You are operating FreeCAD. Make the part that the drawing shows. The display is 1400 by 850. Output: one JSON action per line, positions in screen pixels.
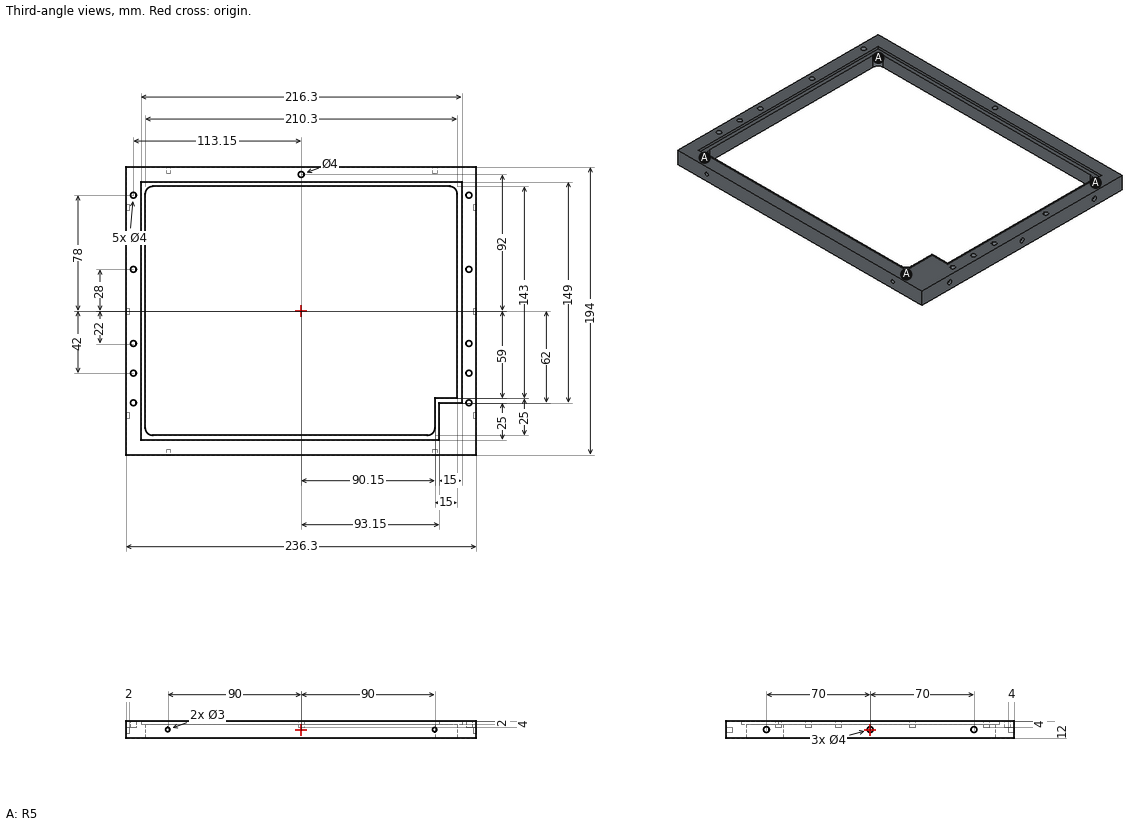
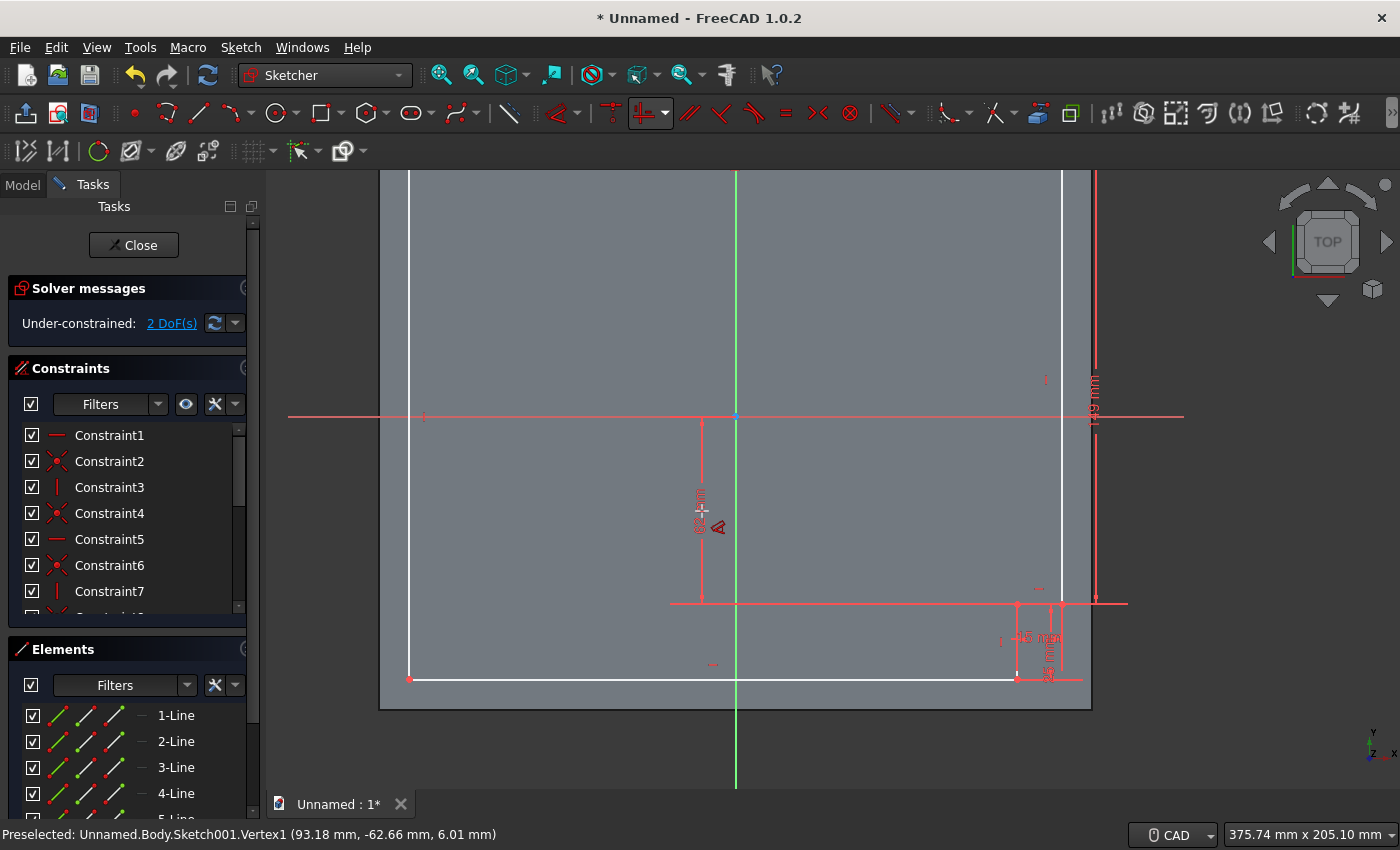
{"action": "scroll", "coordinate": [894, 761], "scroll_direction": "down", "scroll_amount": 1}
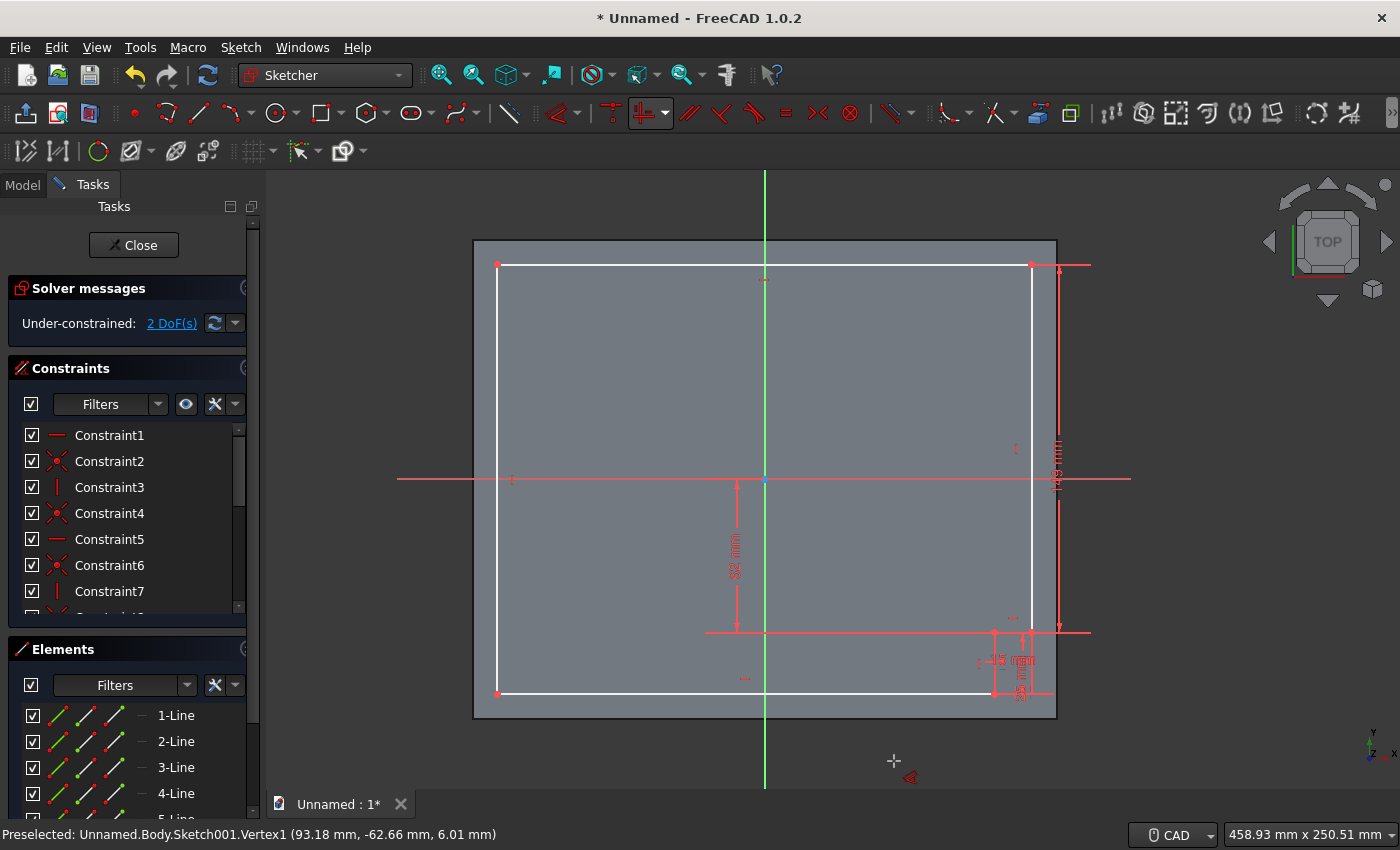
{"action": "left_click", "coordinate": [871, 265]}
{"action": "left_click", "coordinate": [641, 231]}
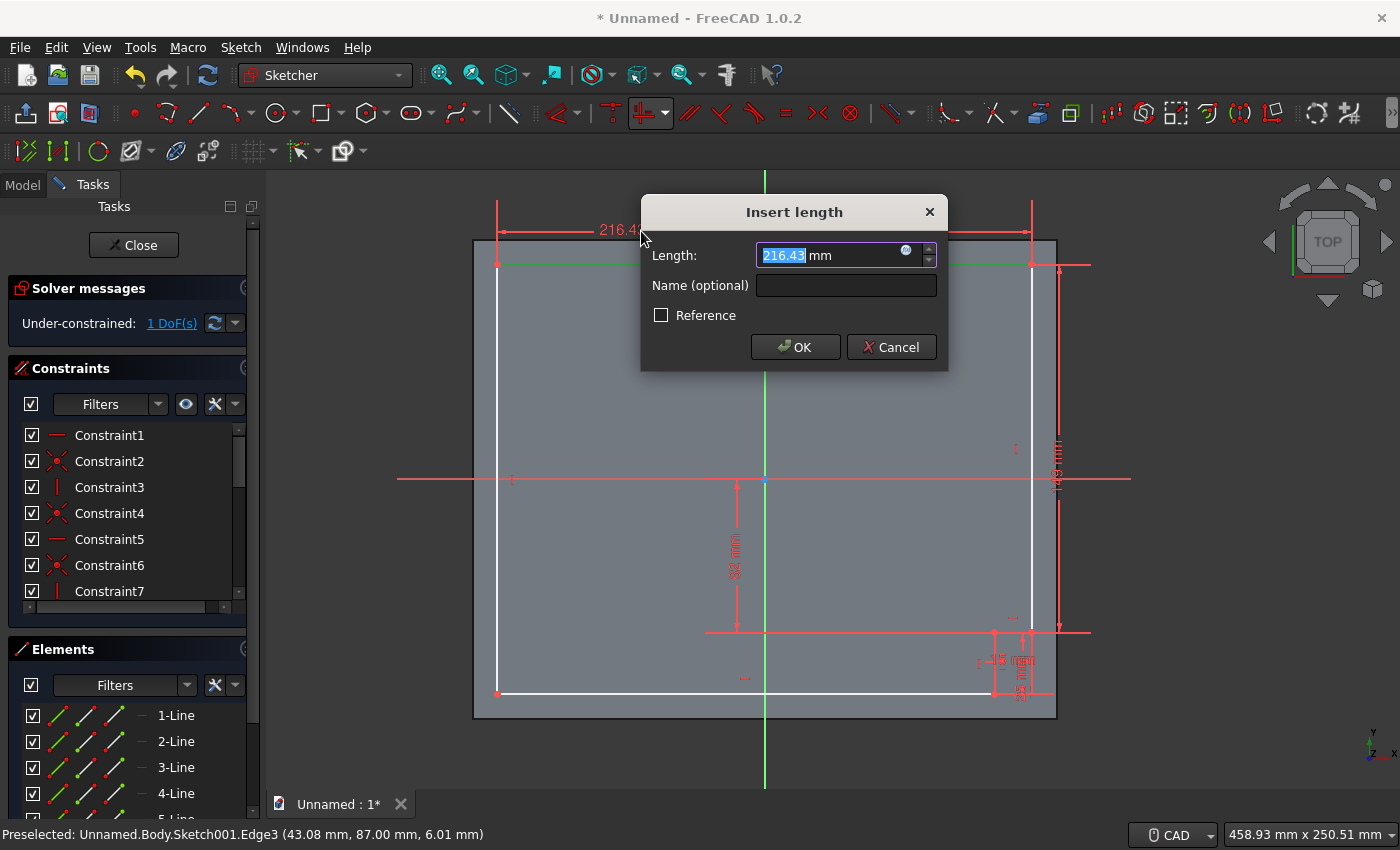
{"action": "type", "text": "216.3"}
{"action": "key", "text": "Return"}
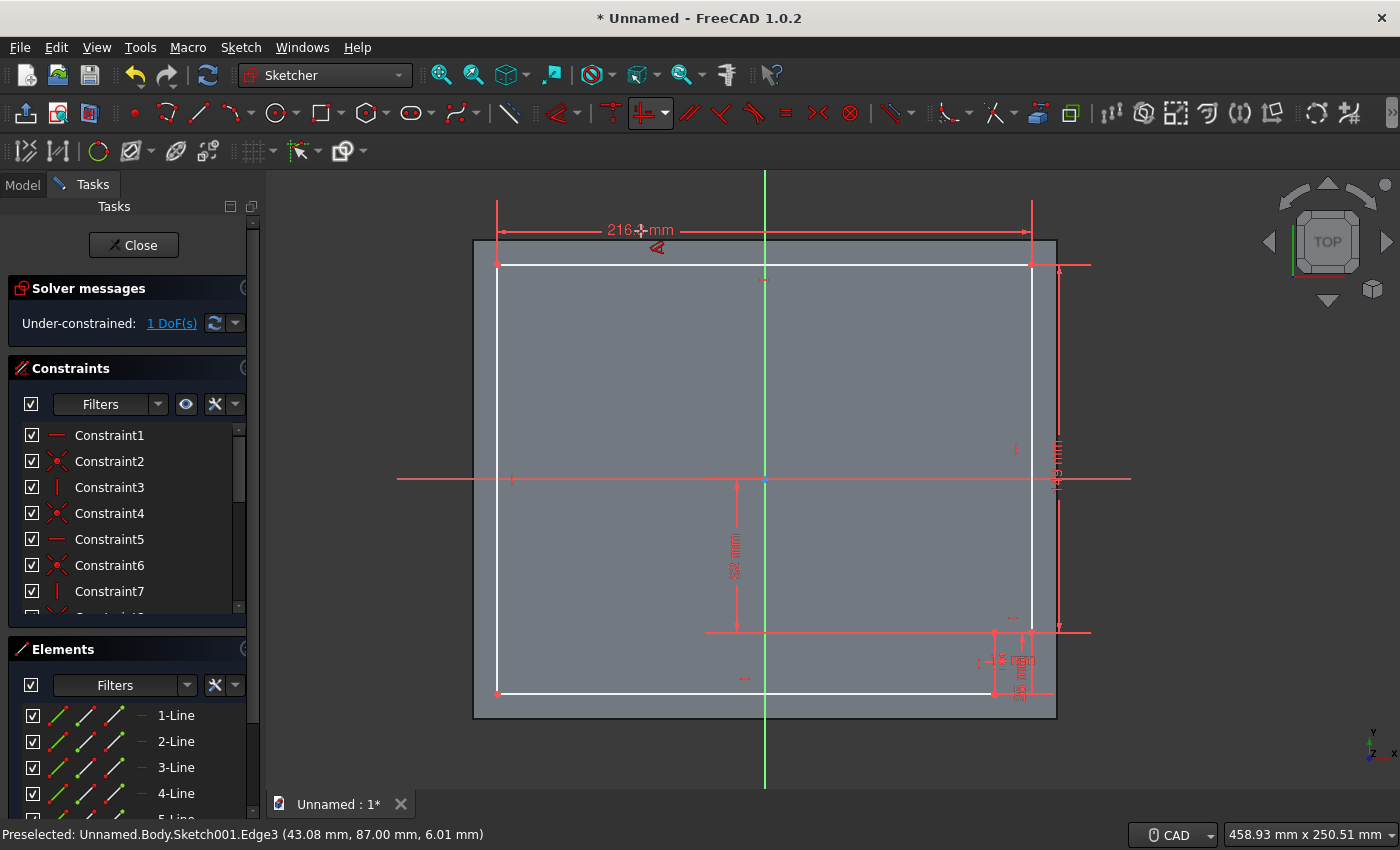
{"action": "left_click", "coordinate": [995, 633]}
{"action": "left_click", "coordinate": [880, 667]}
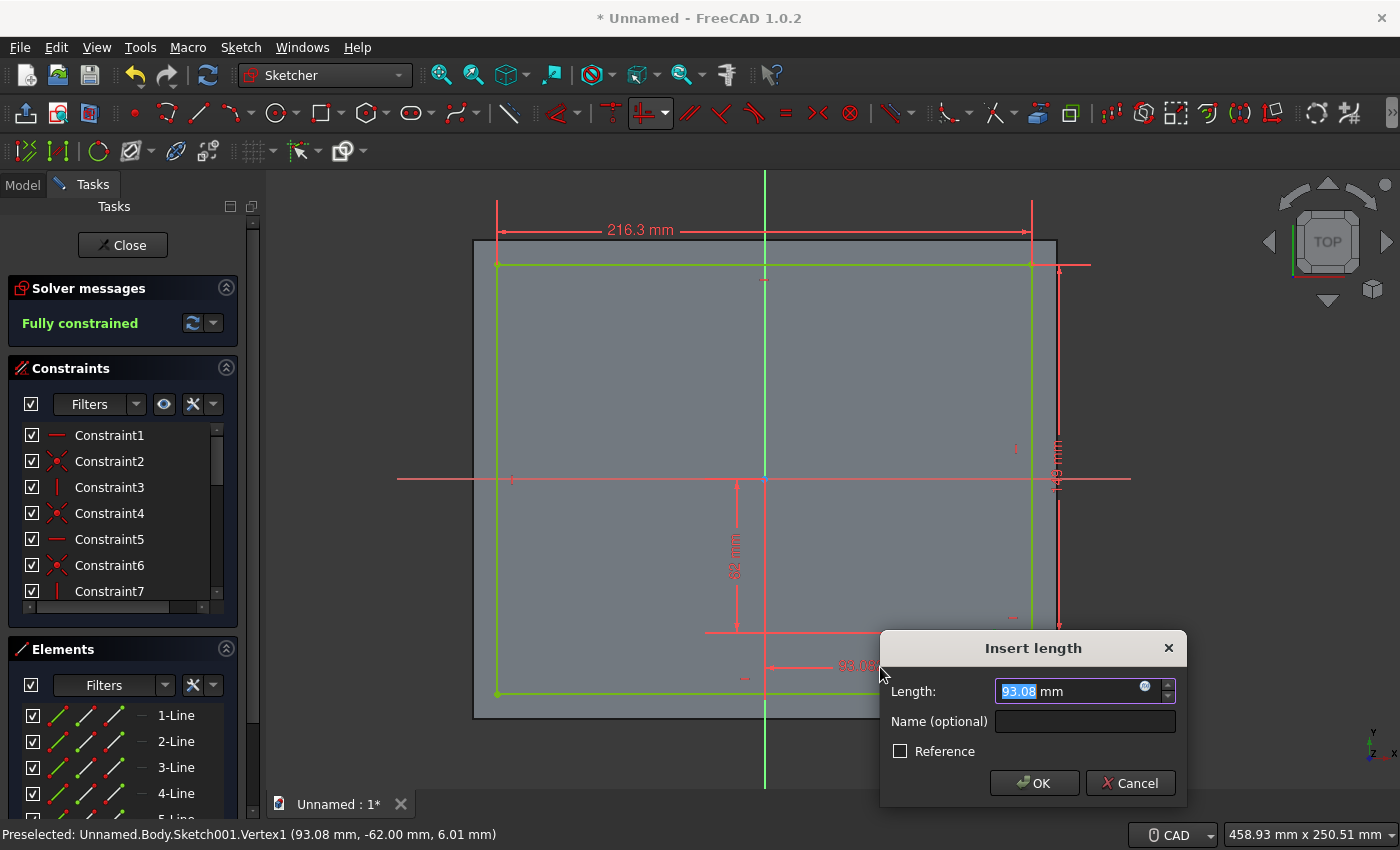
{"action": "type", "text": "93.15"}
{"action": "key", "text": "Return"}
{"action": "key", "text": "Escape"}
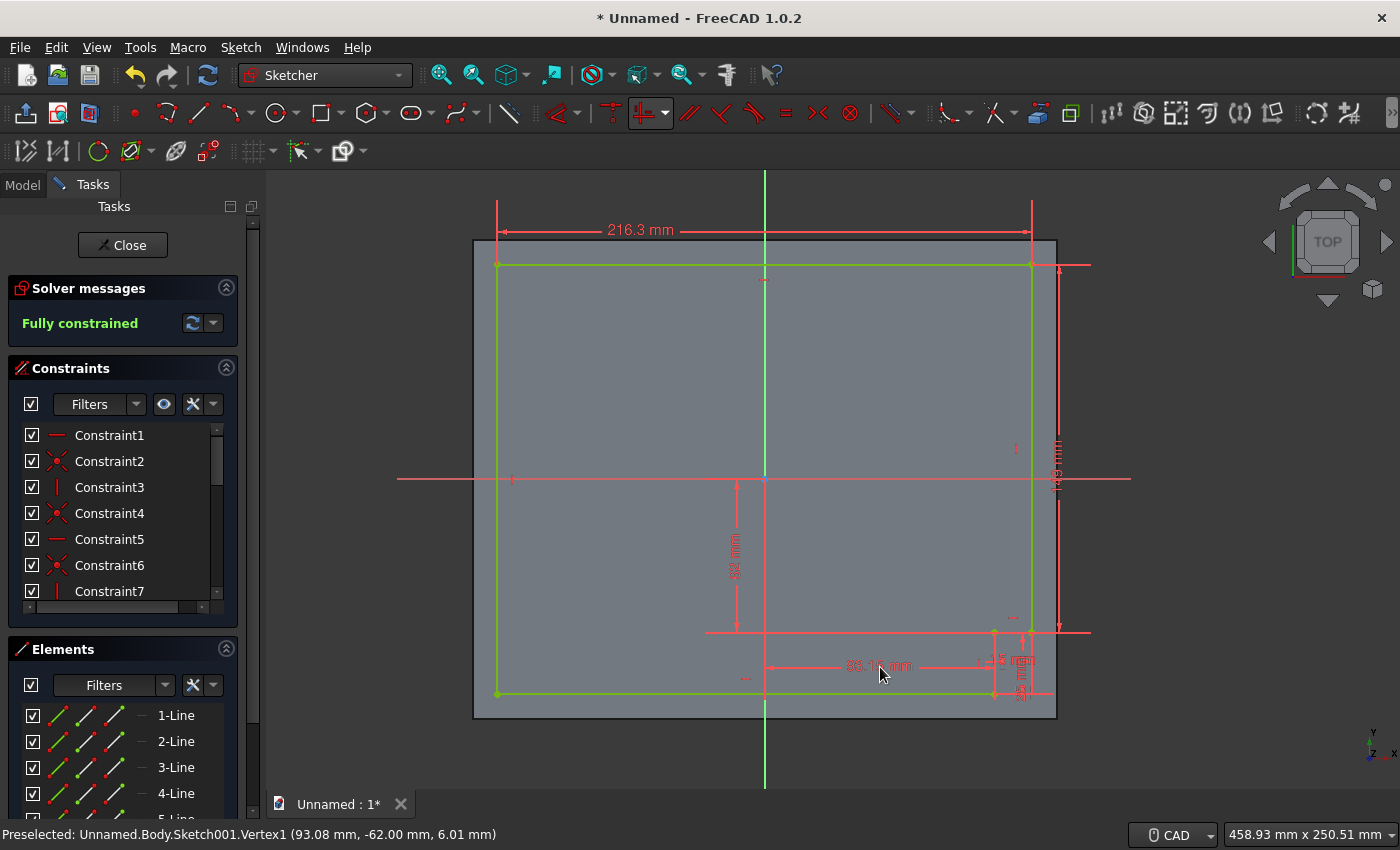
{"action": "left_click", "coordinate": [123, 245]}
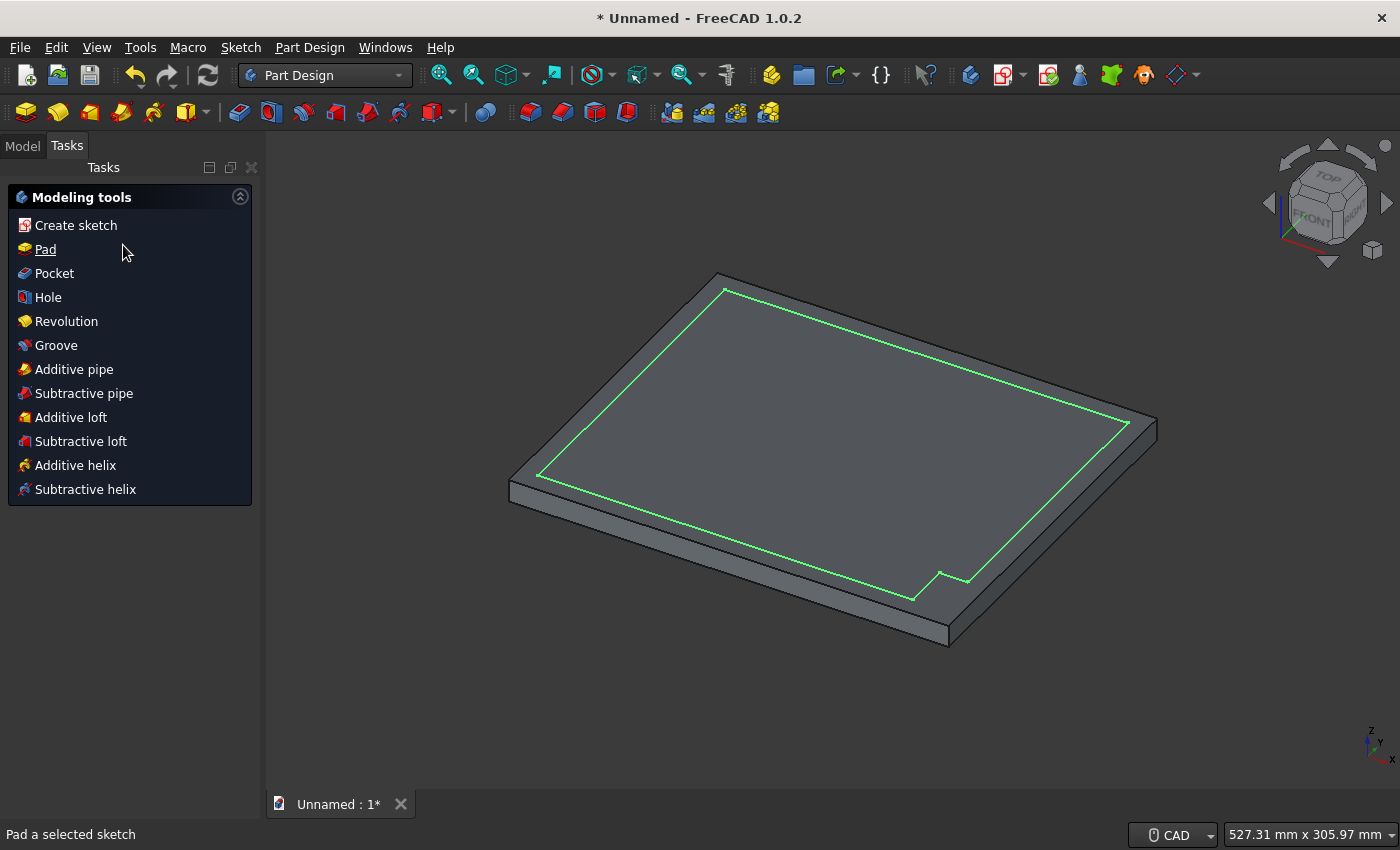
{"action": "left_click", "coordinate": [240, 112]}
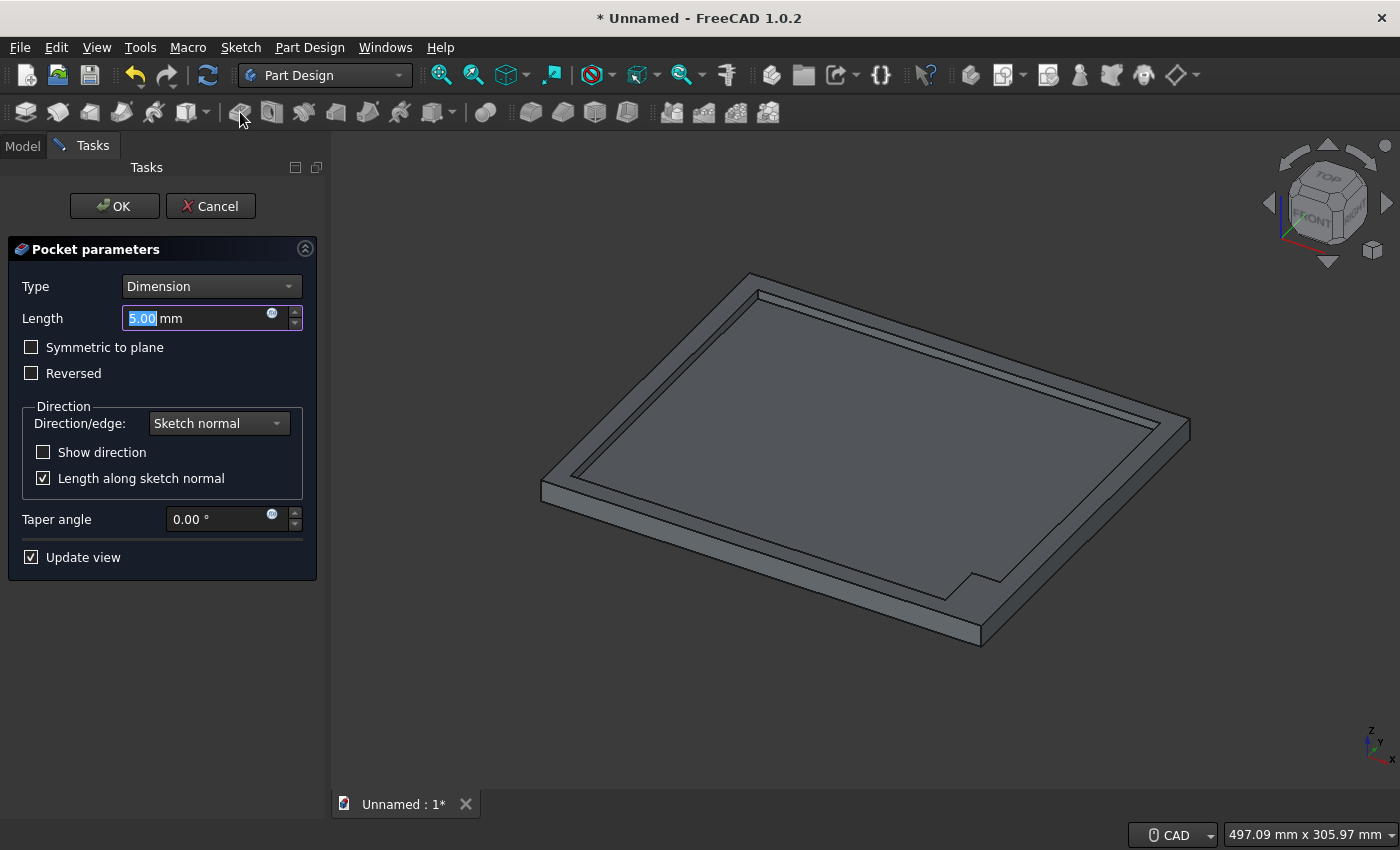
{"action": "type", "text": "2"}
{"action": "key", "text": "Tab"}